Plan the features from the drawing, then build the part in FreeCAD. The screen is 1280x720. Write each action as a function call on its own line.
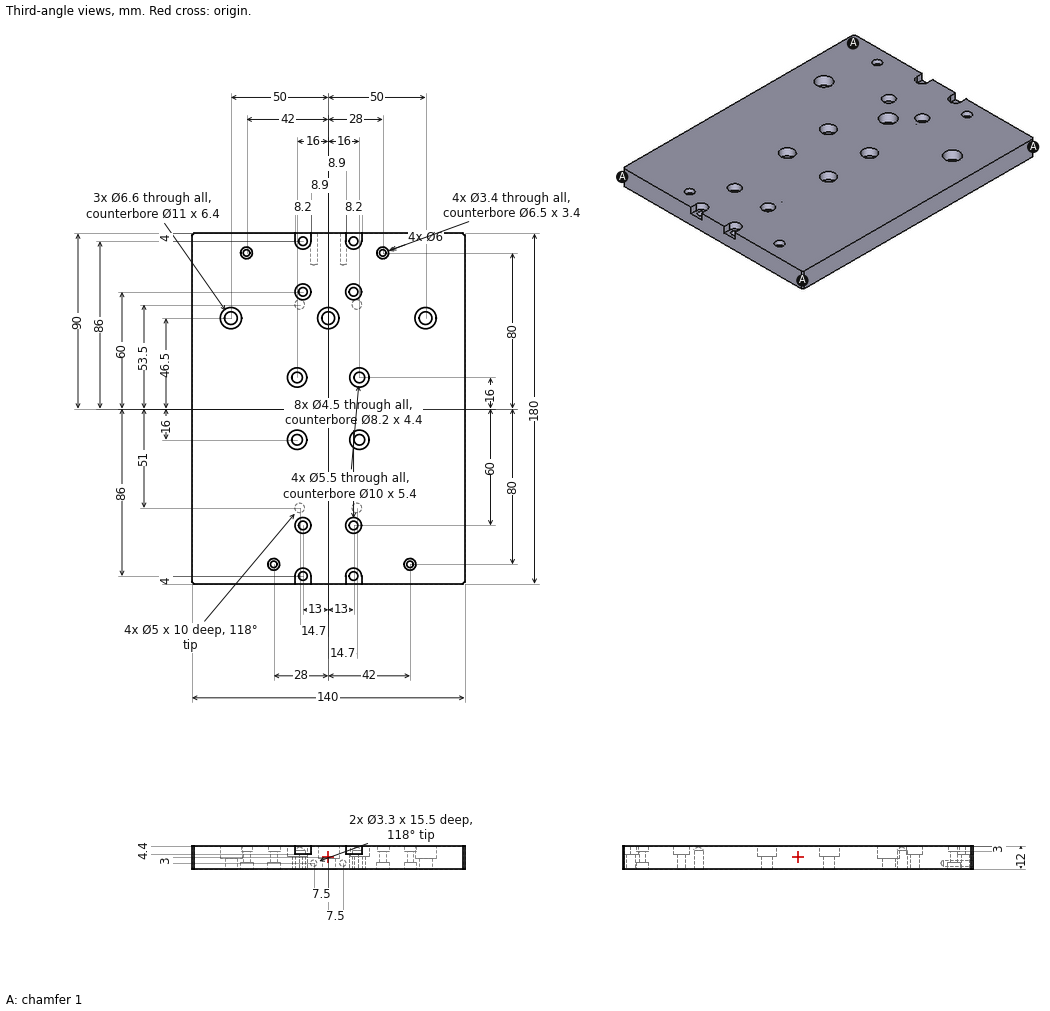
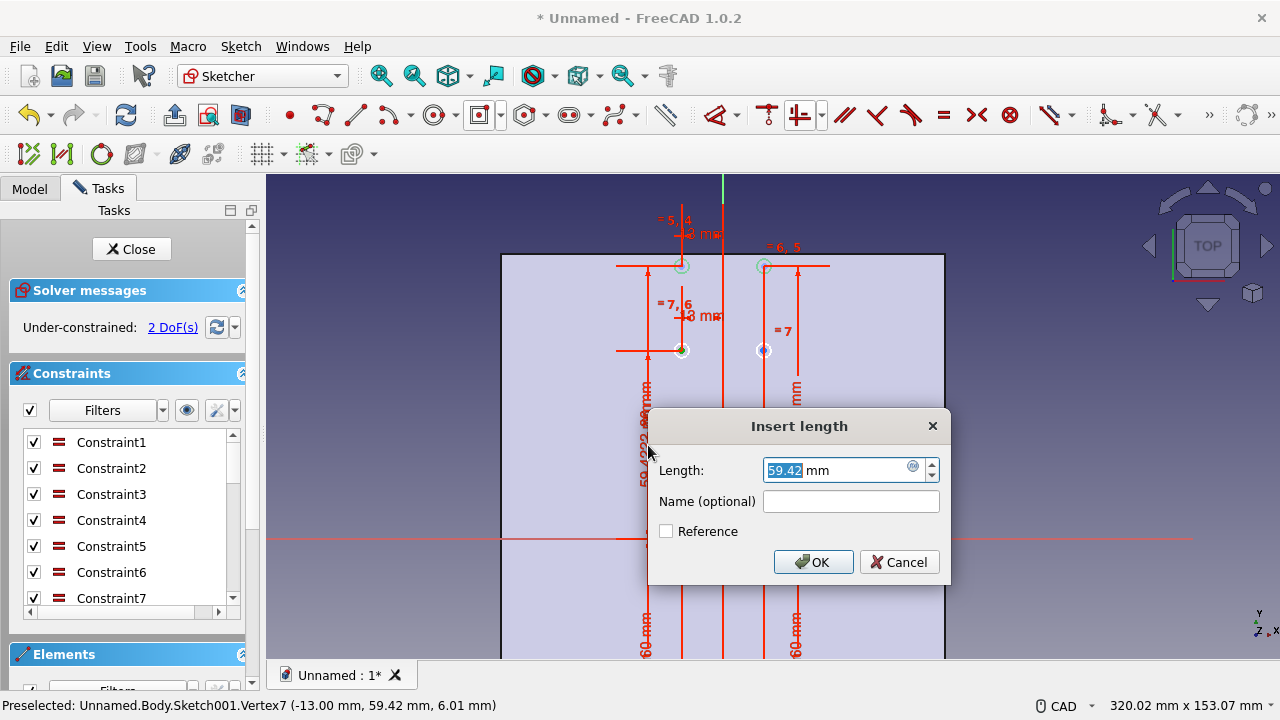
text(60)
key(Return)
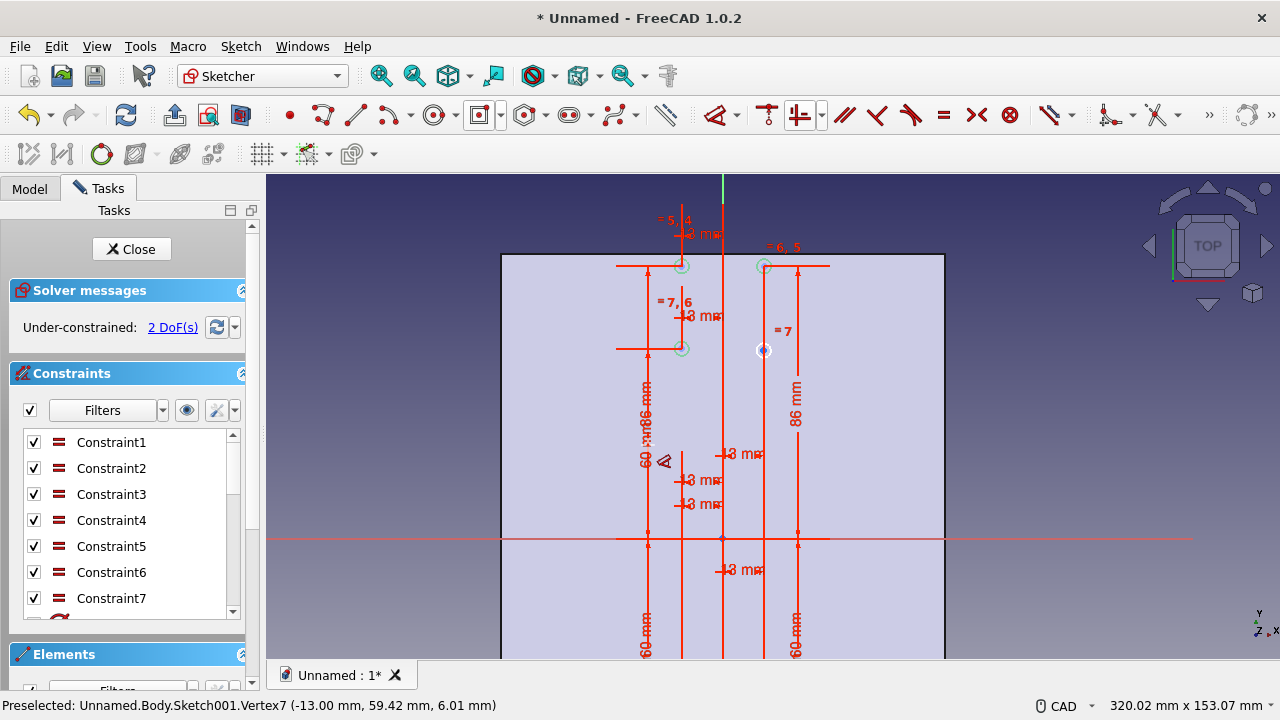
click(764, 351)
click(743, 293)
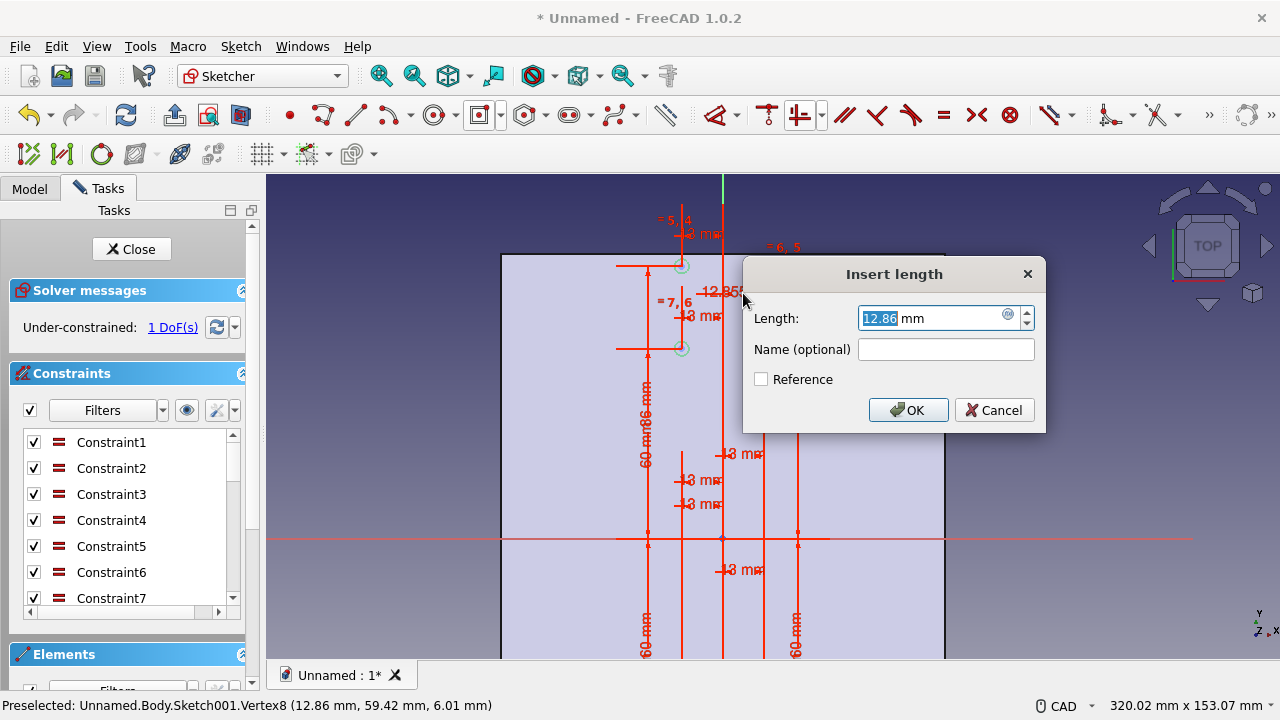
text(13)
key(Return)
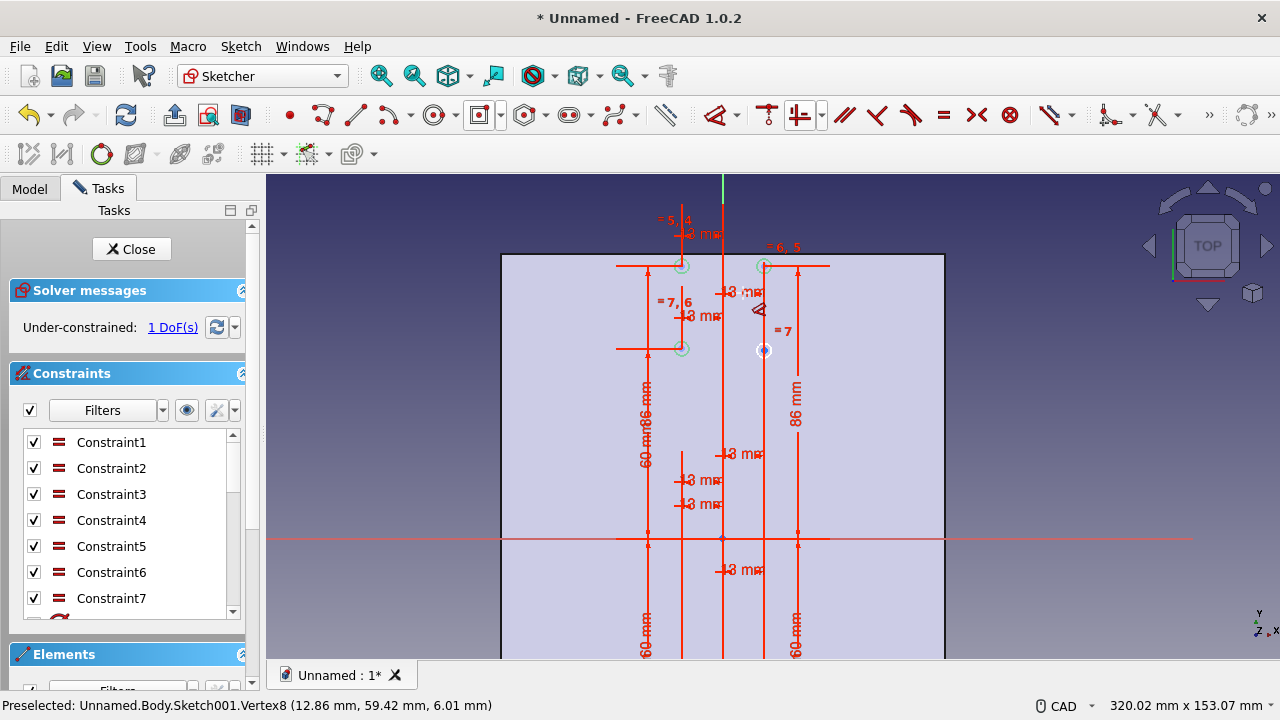
click(764, 351)
click(798, 488)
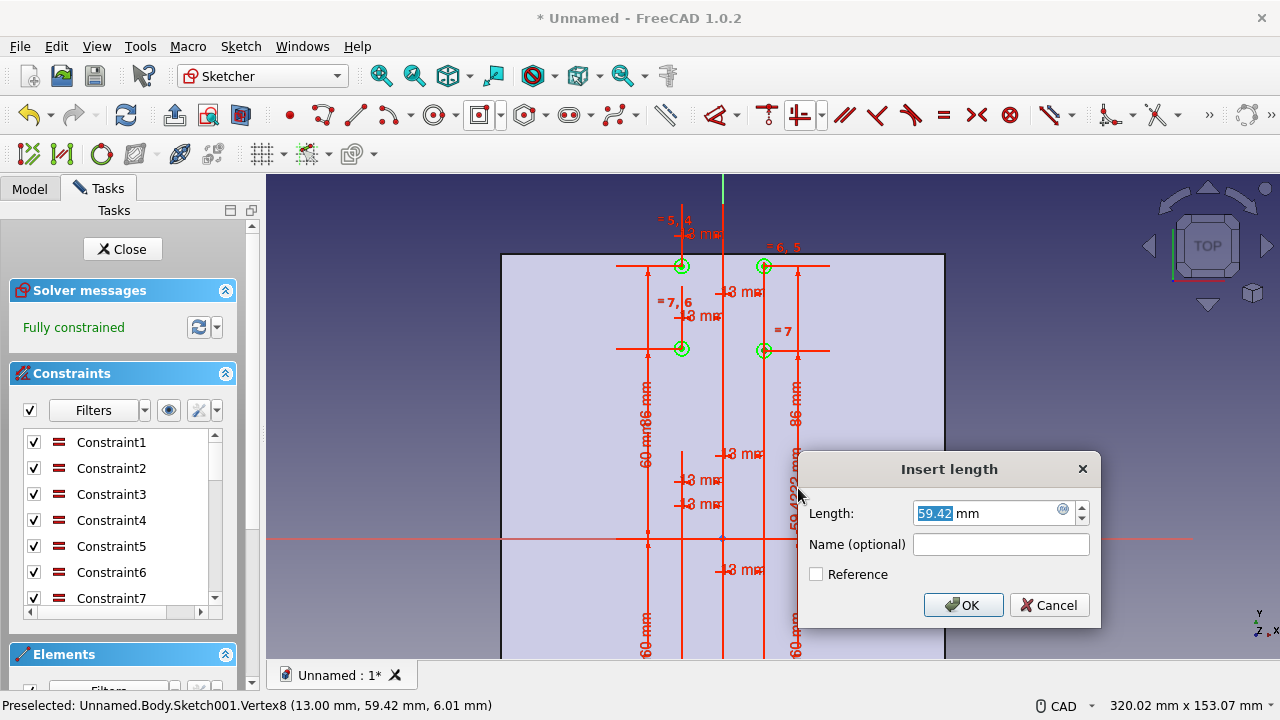
text(60)
key(Return)
key(Escape)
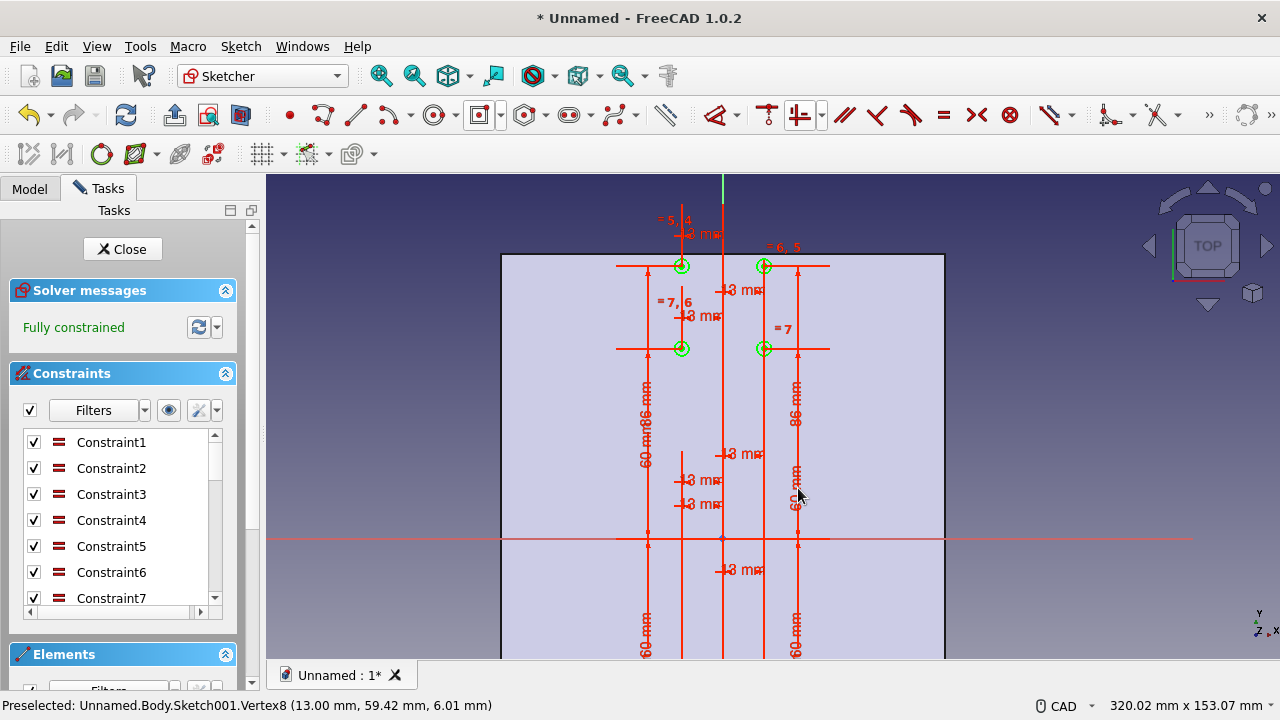
click(123, 249)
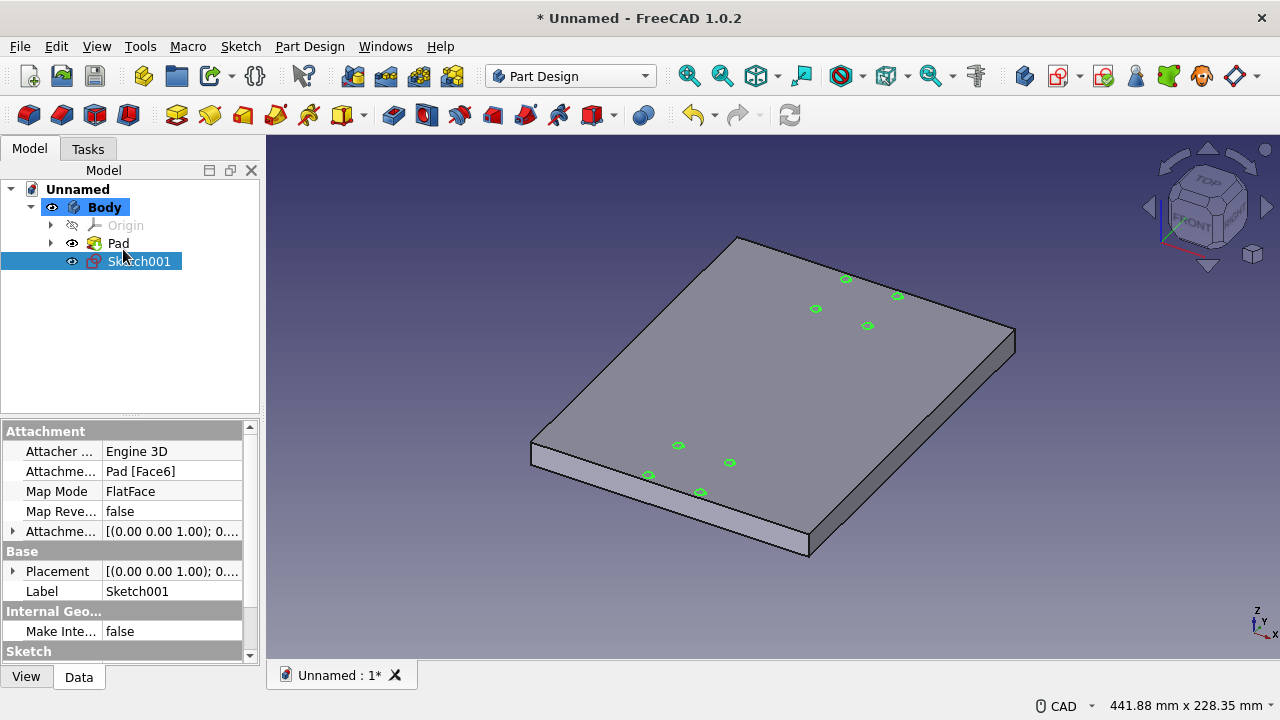
click(427, 116)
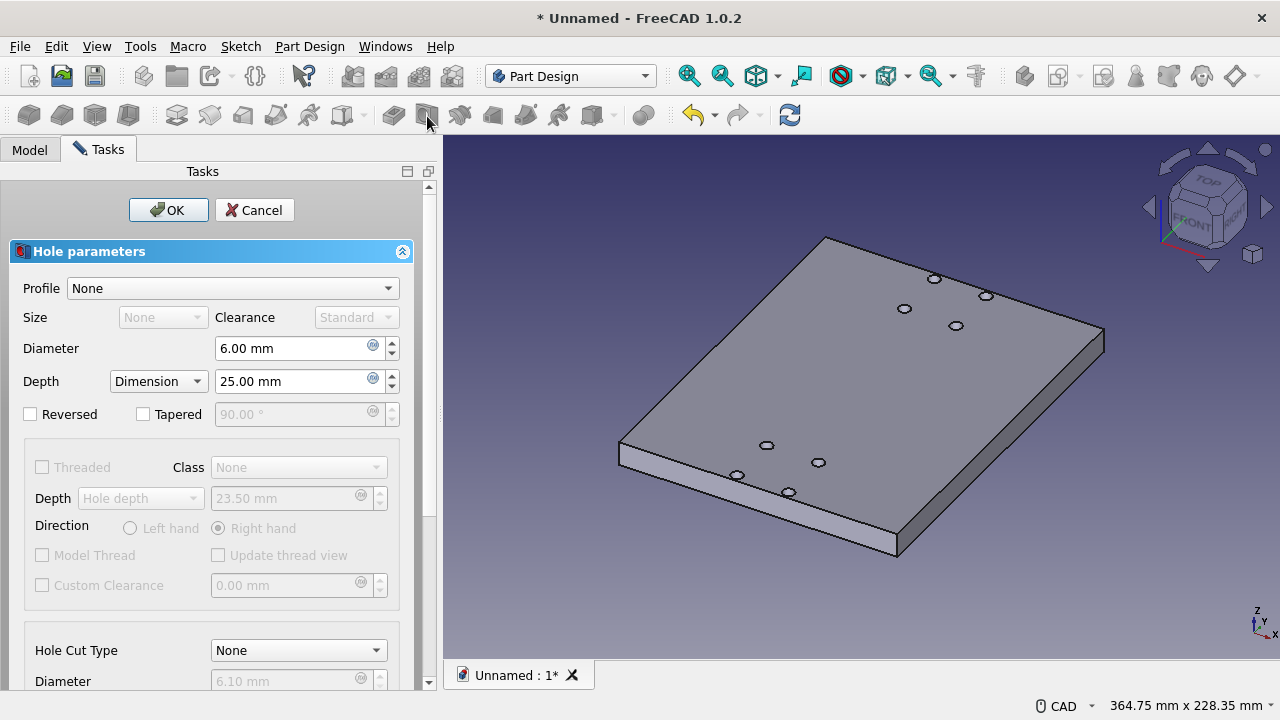
triple_click(300, 348)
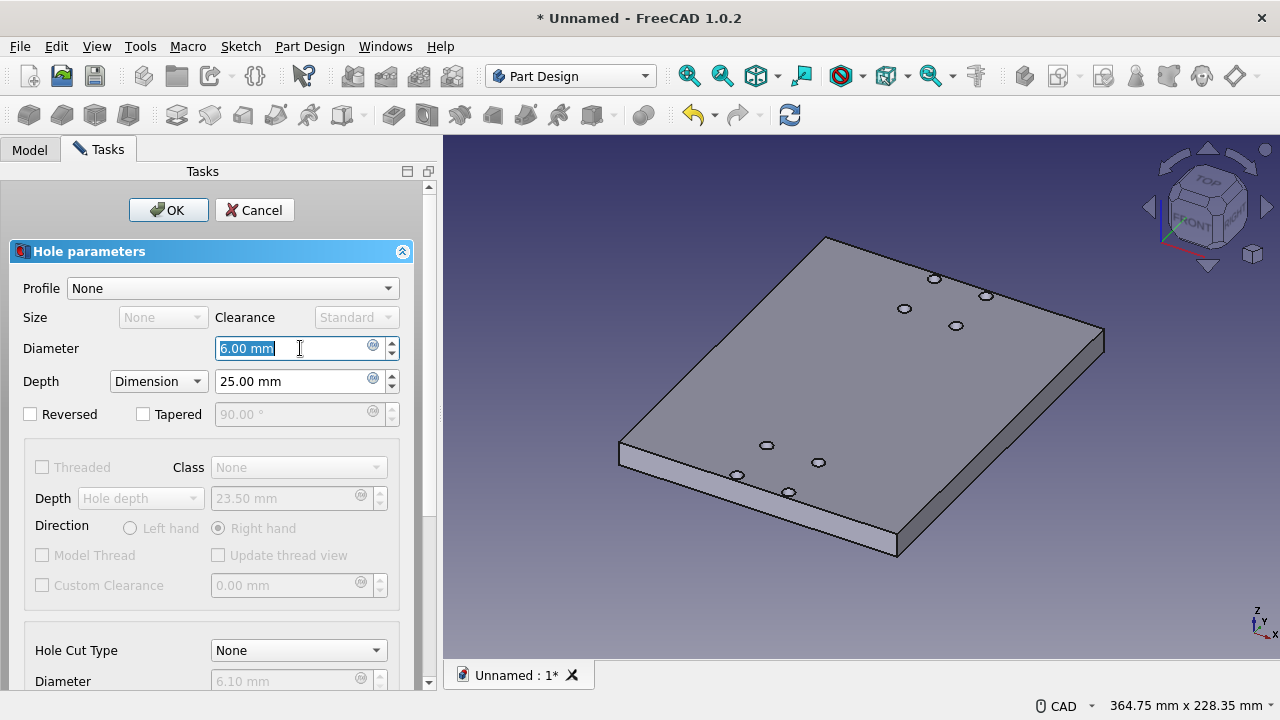
text(4.5)
key(Tab)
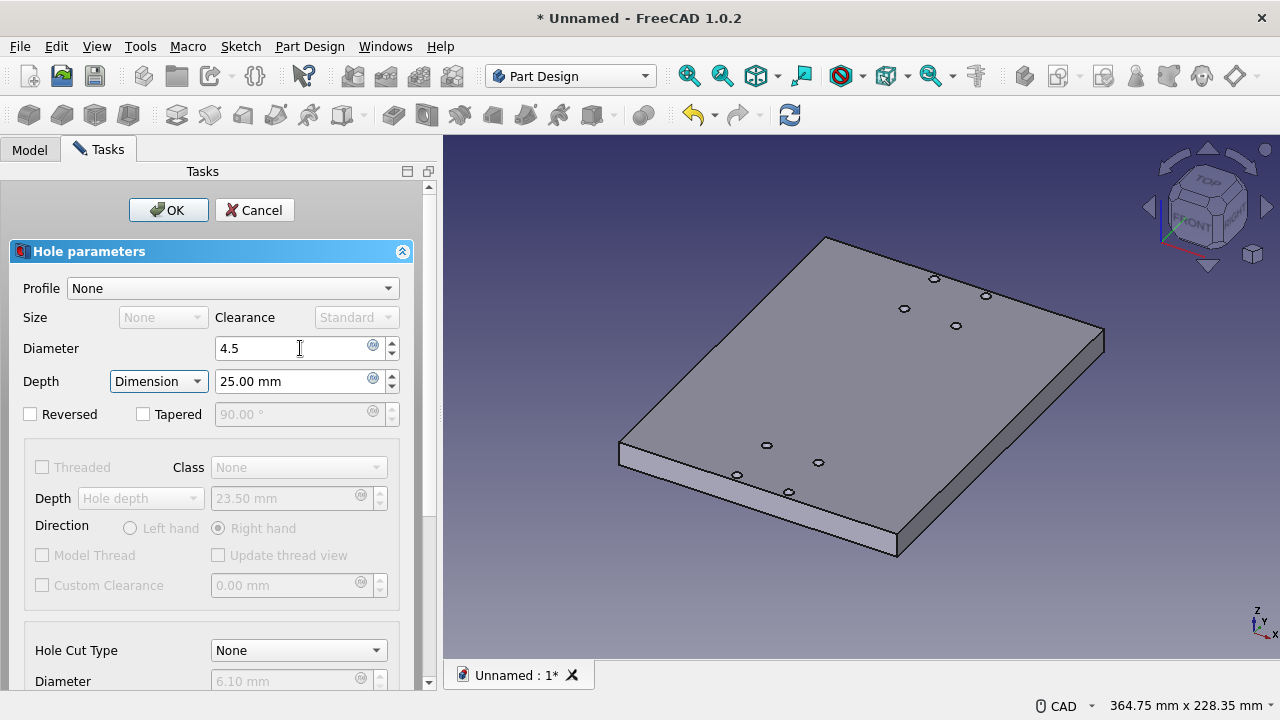
click(160, 382)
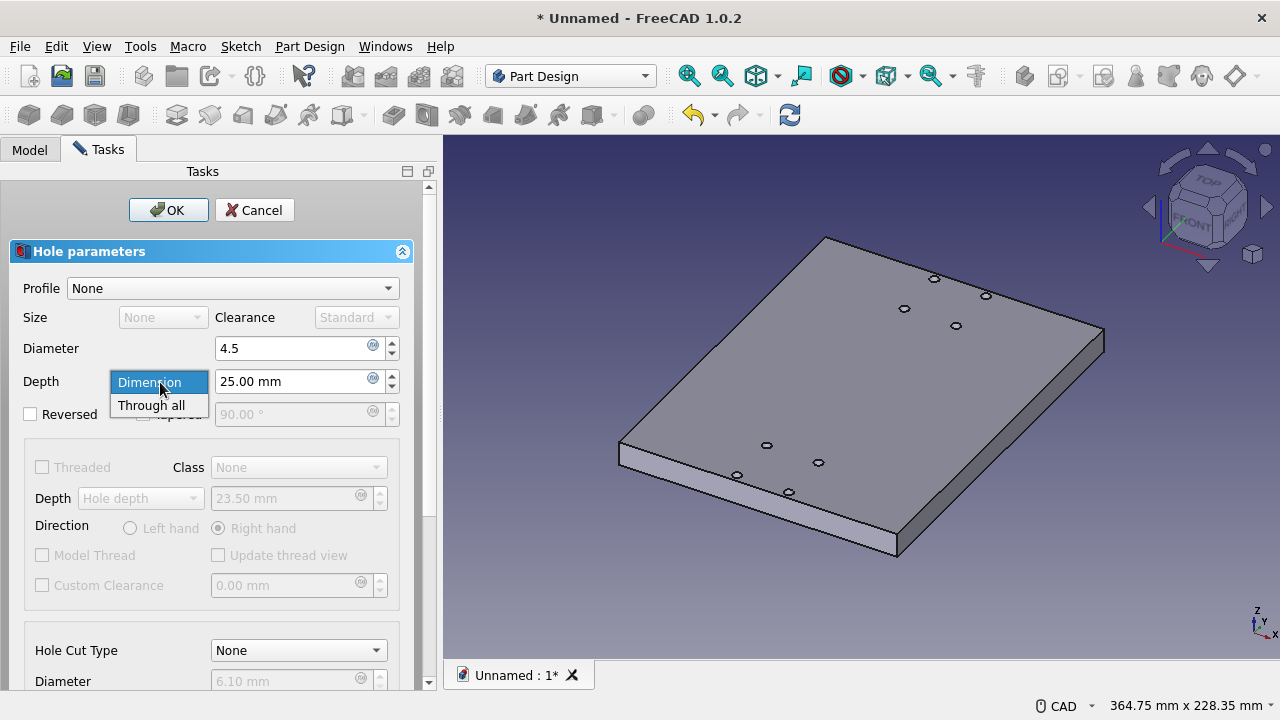
click(158, 406)